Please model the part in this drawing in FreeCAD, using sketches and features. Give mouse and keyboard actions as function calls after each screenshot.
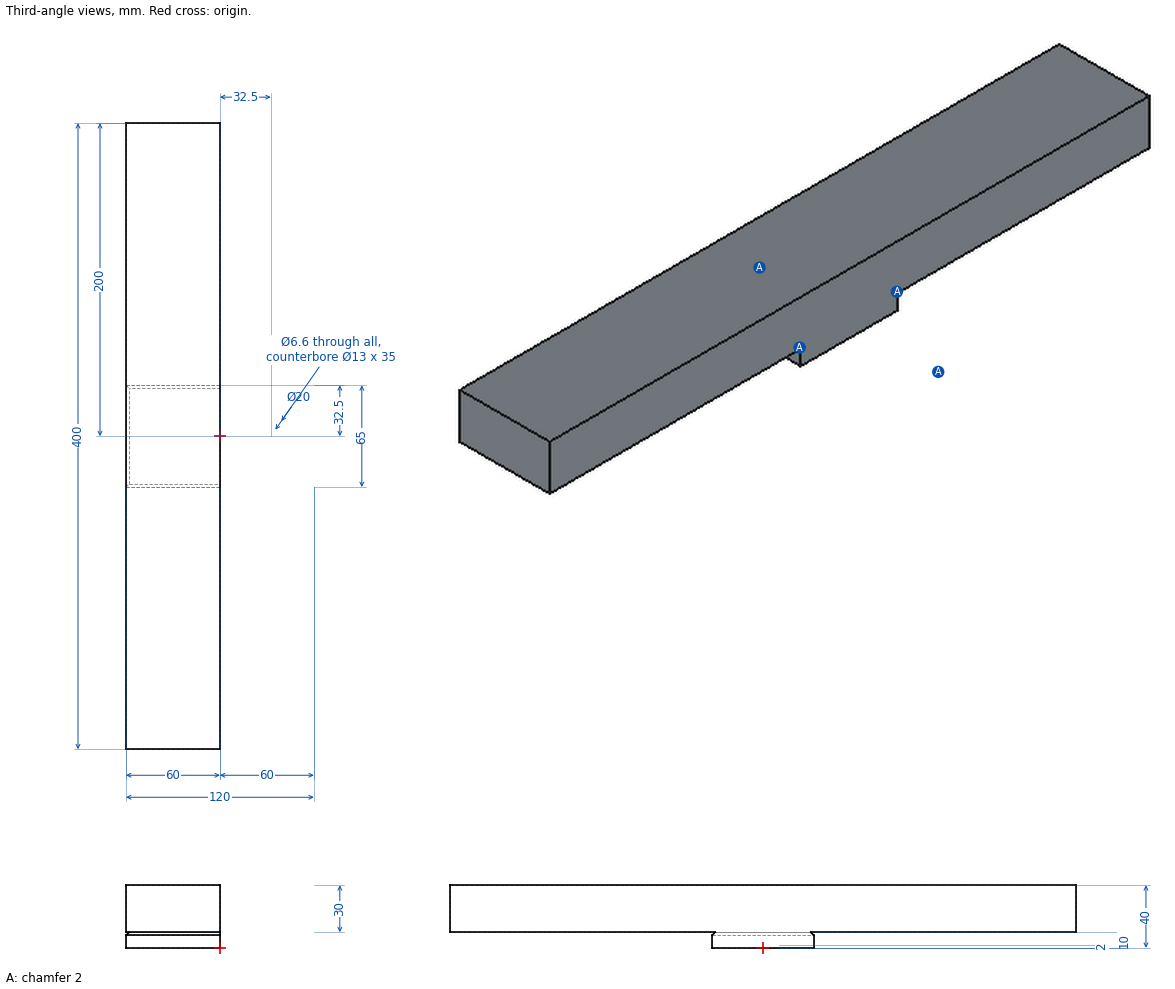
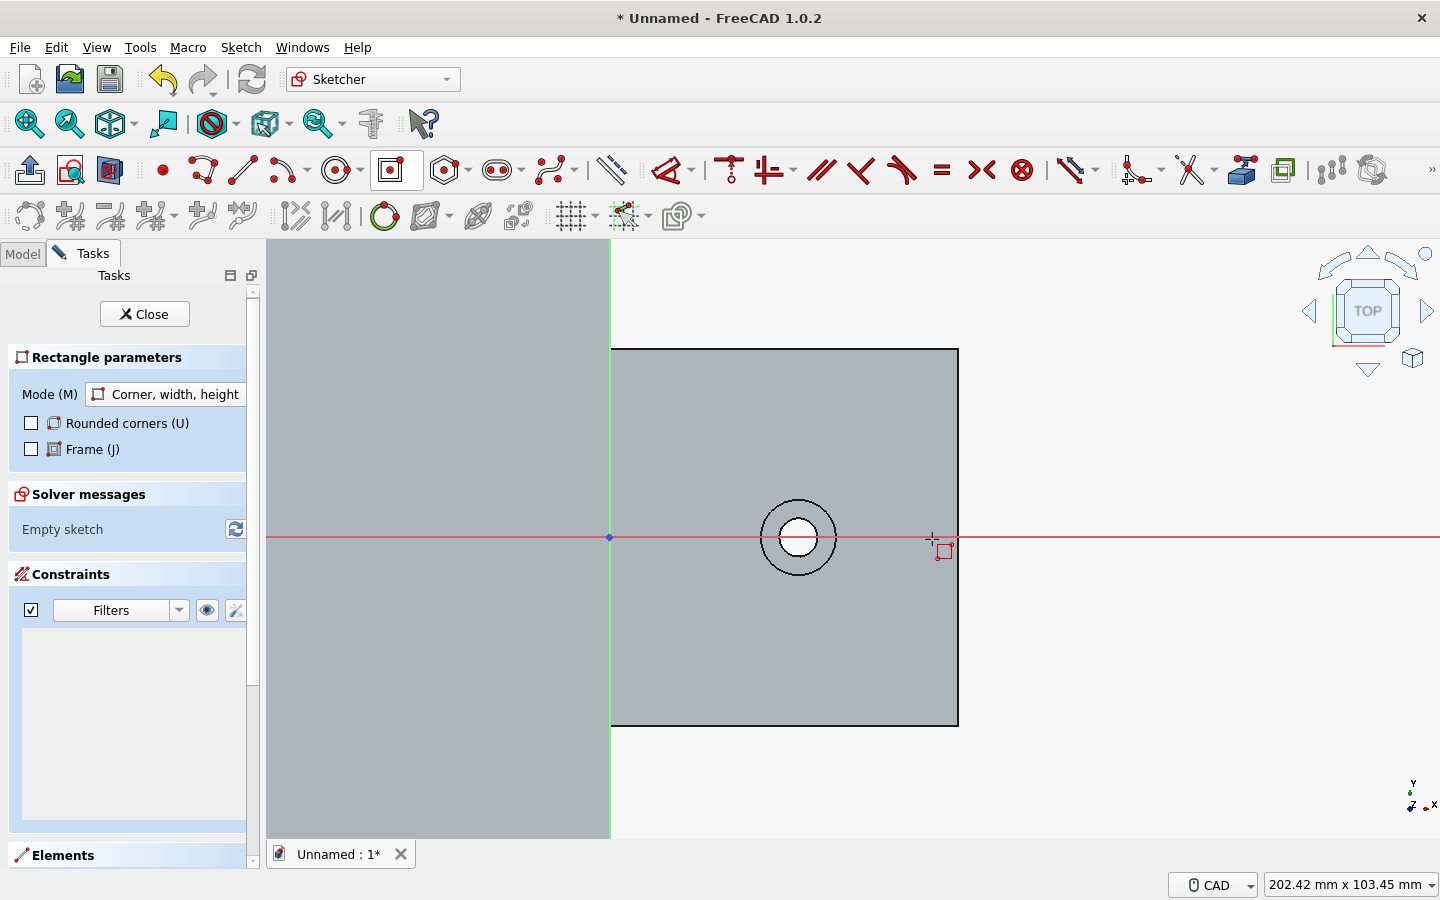
click(610, 349)
click(958, 726)
key(Escape)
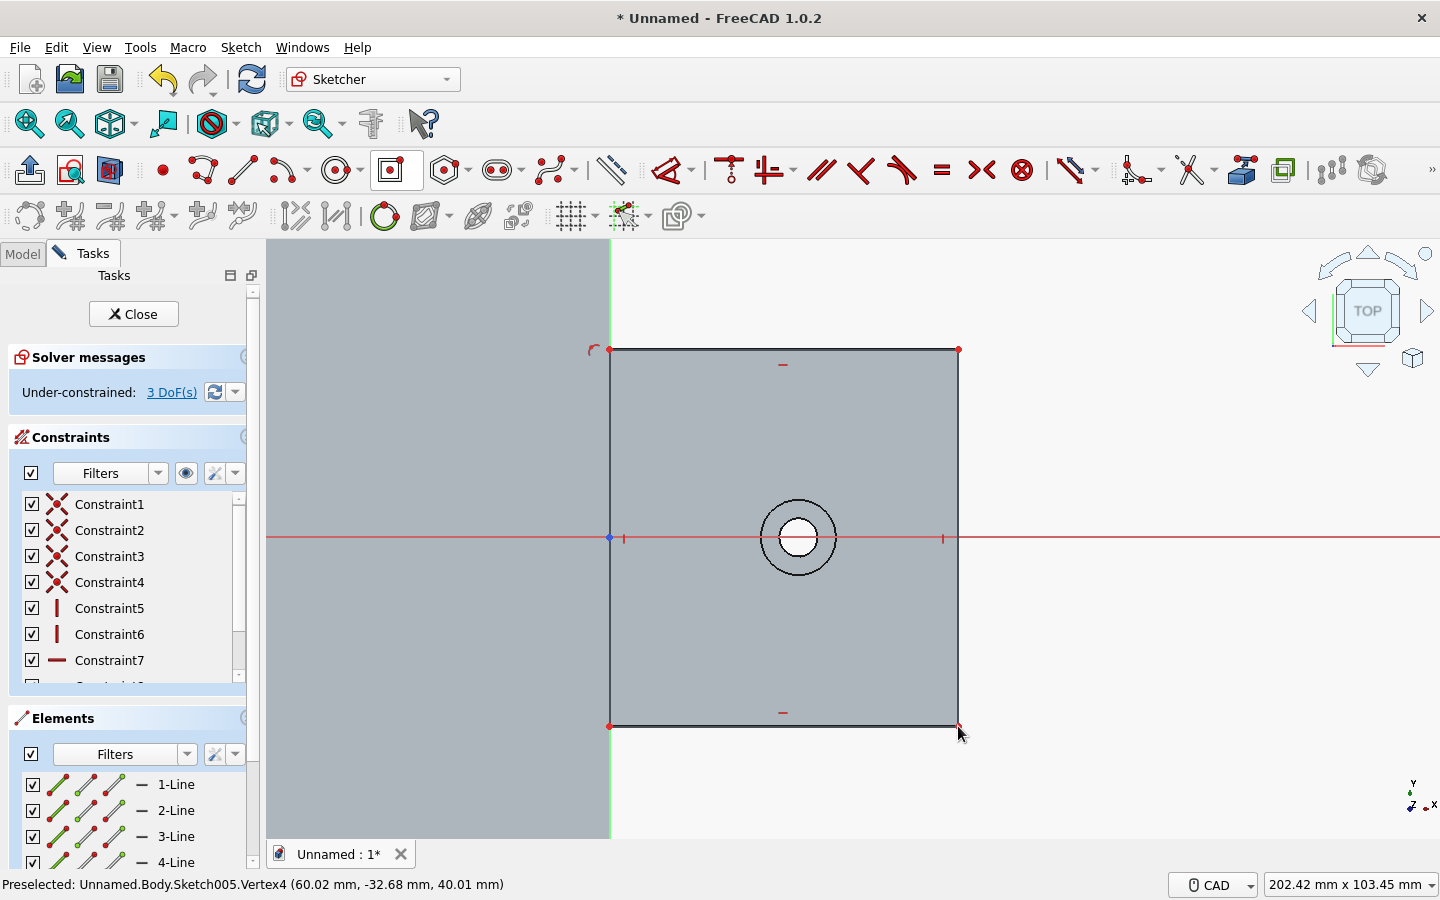
click(666, 170)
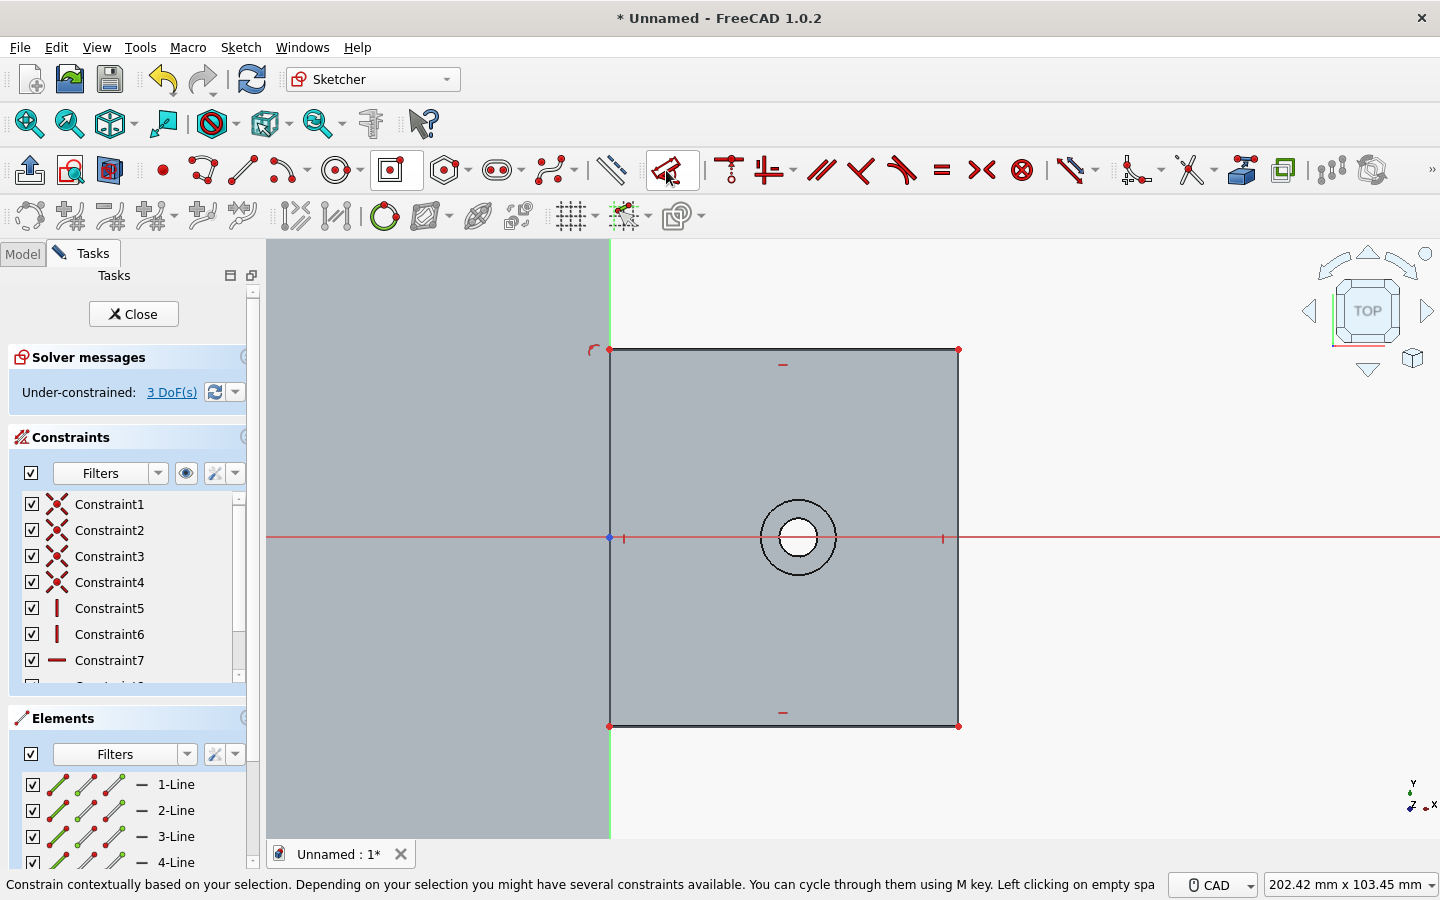
click(610, 463)
click(576, 452)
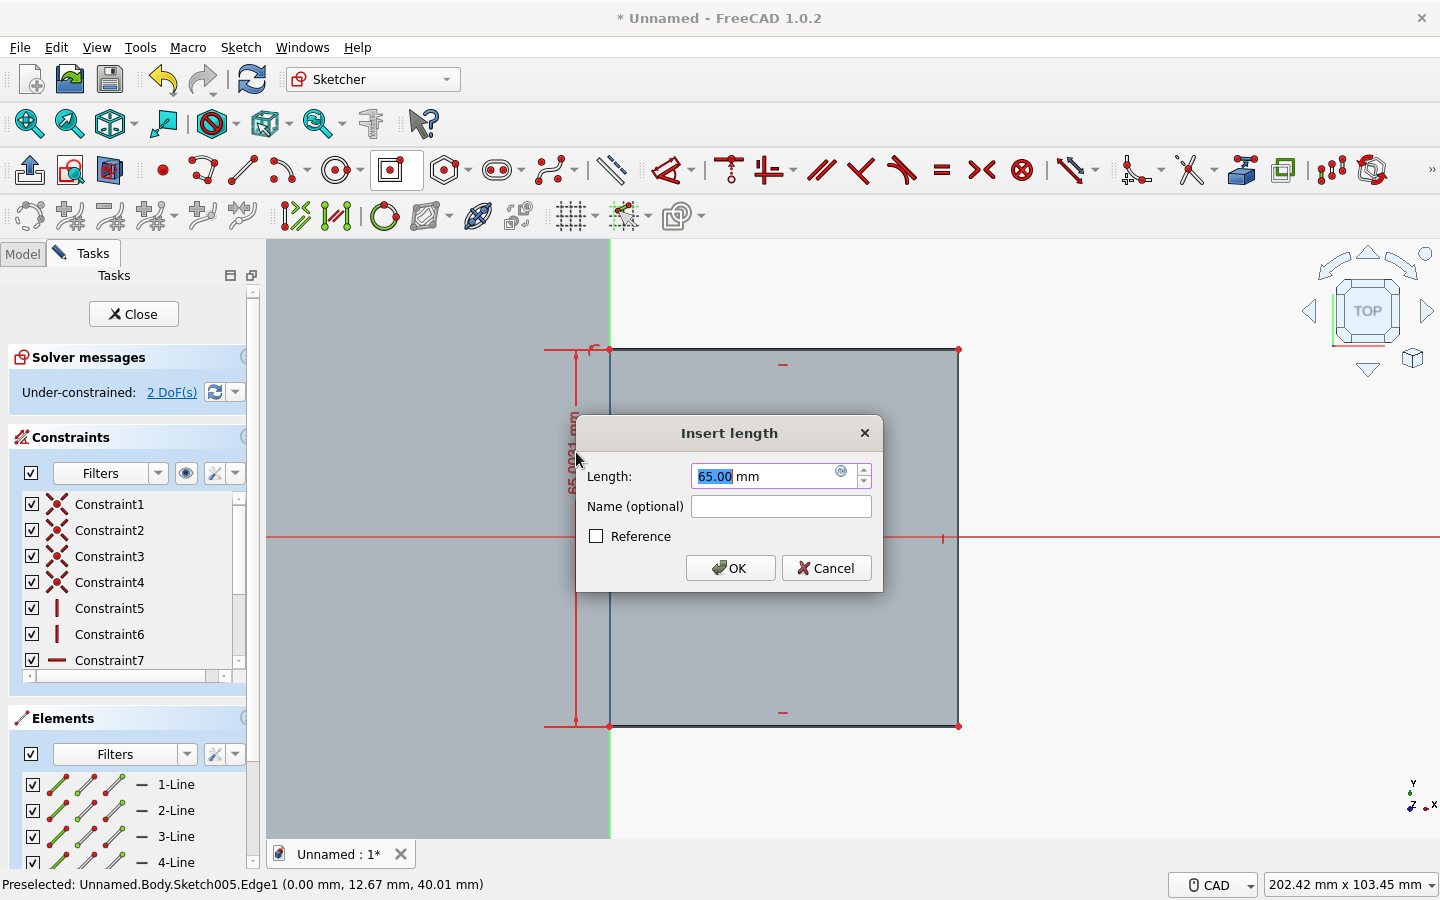
text(65)
key(Return)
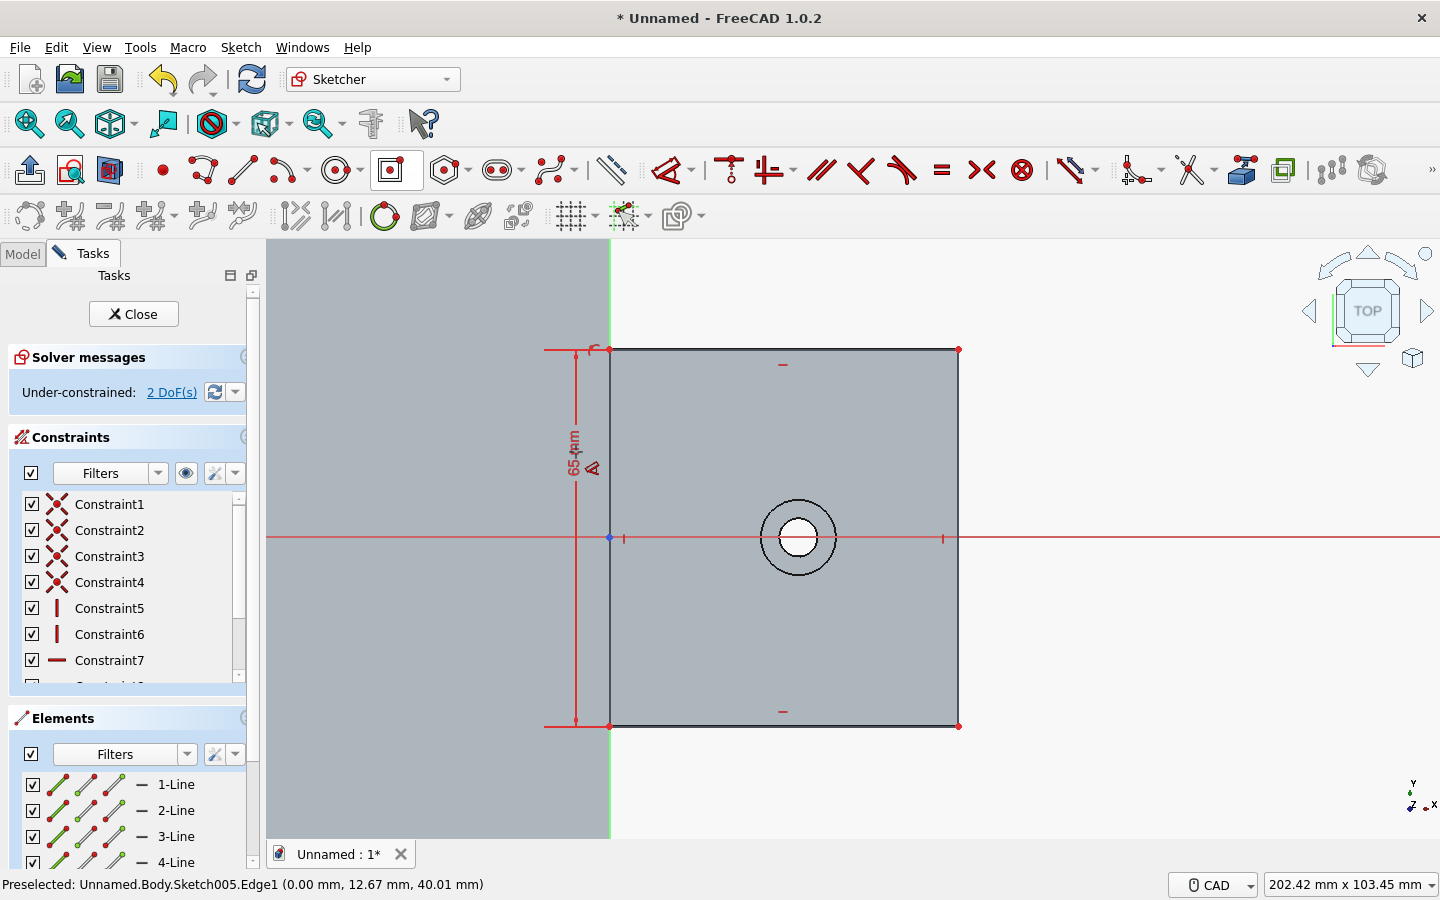
click(714, 727)
click(784, 761)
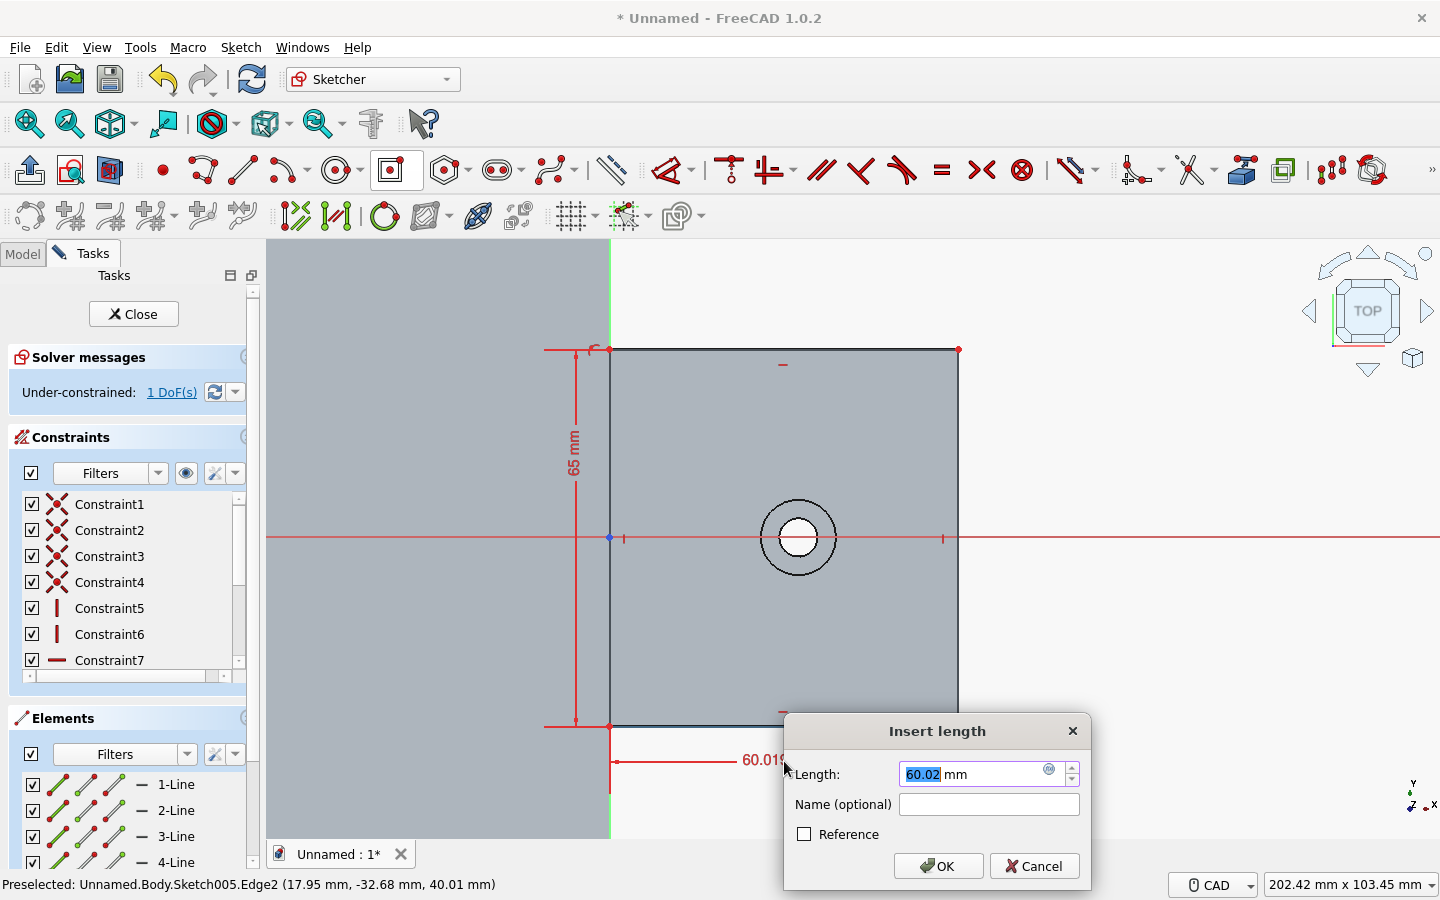
text(60)
key(Return)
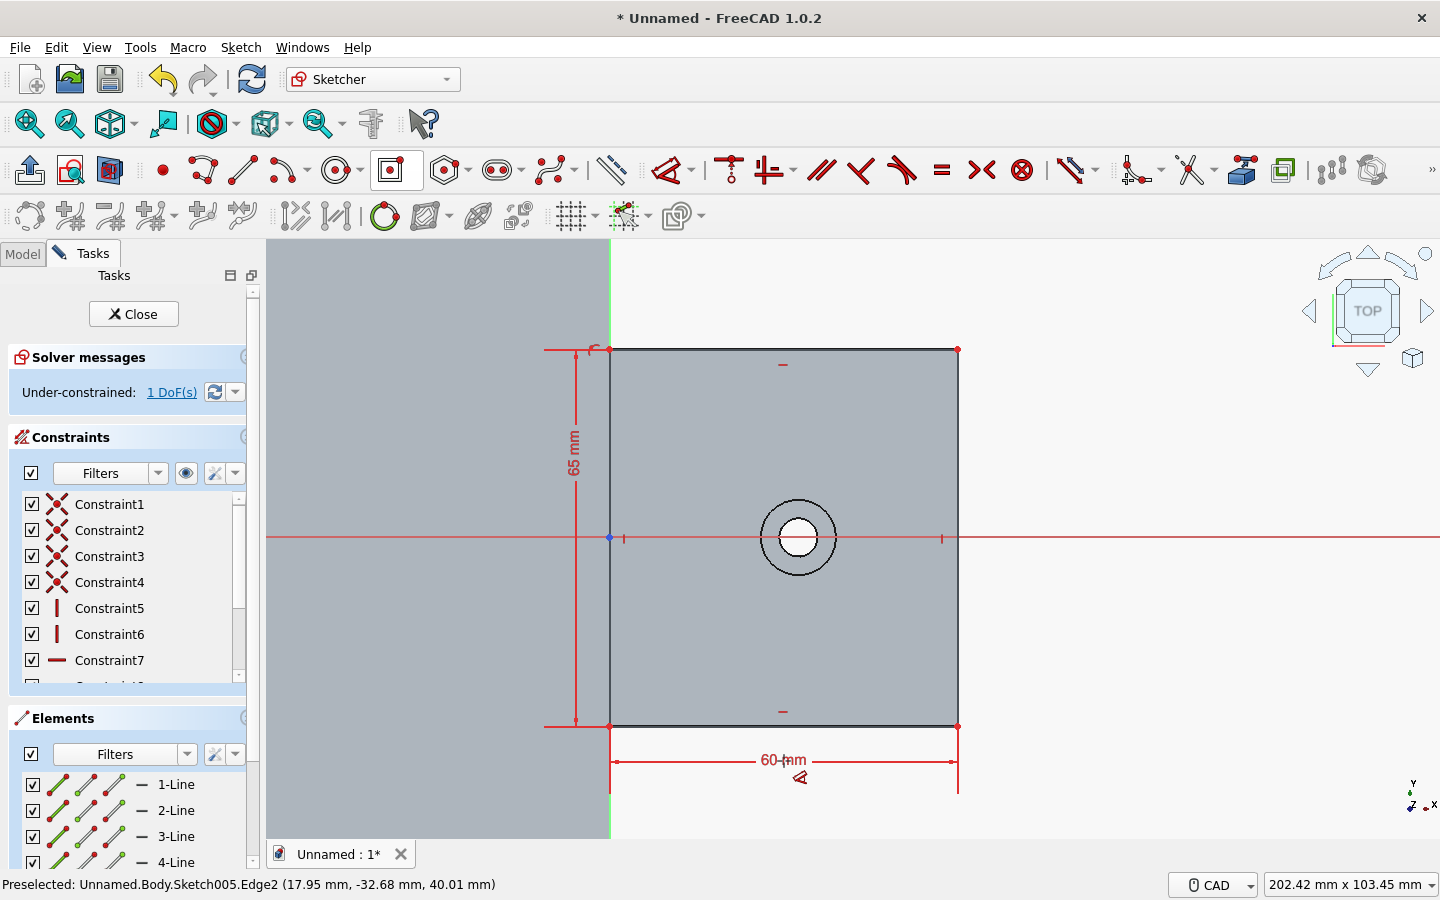
click(610, 350)
click(576, 401)